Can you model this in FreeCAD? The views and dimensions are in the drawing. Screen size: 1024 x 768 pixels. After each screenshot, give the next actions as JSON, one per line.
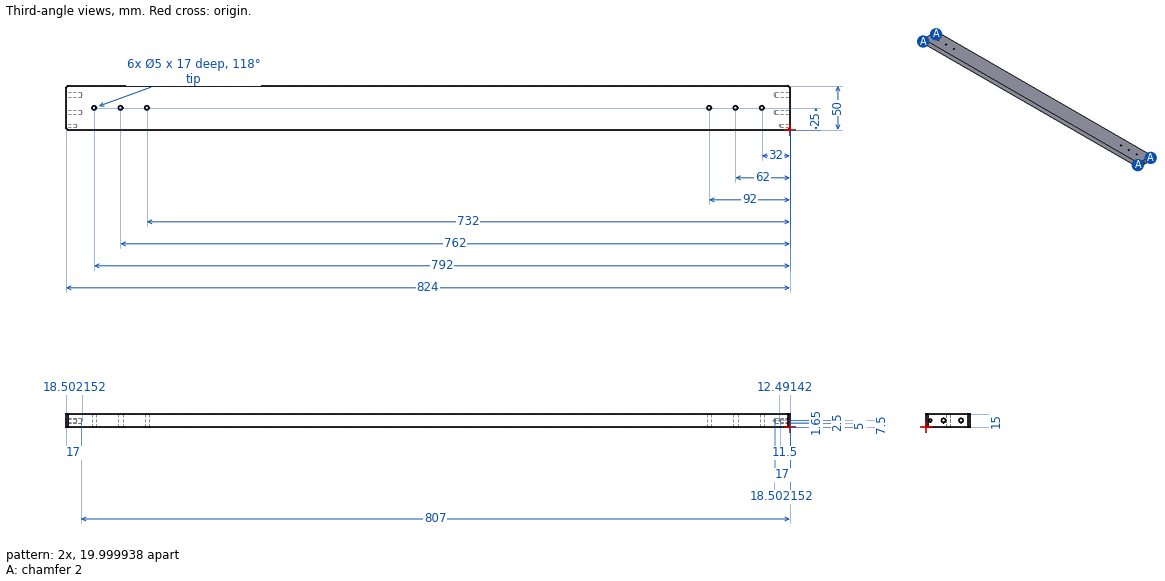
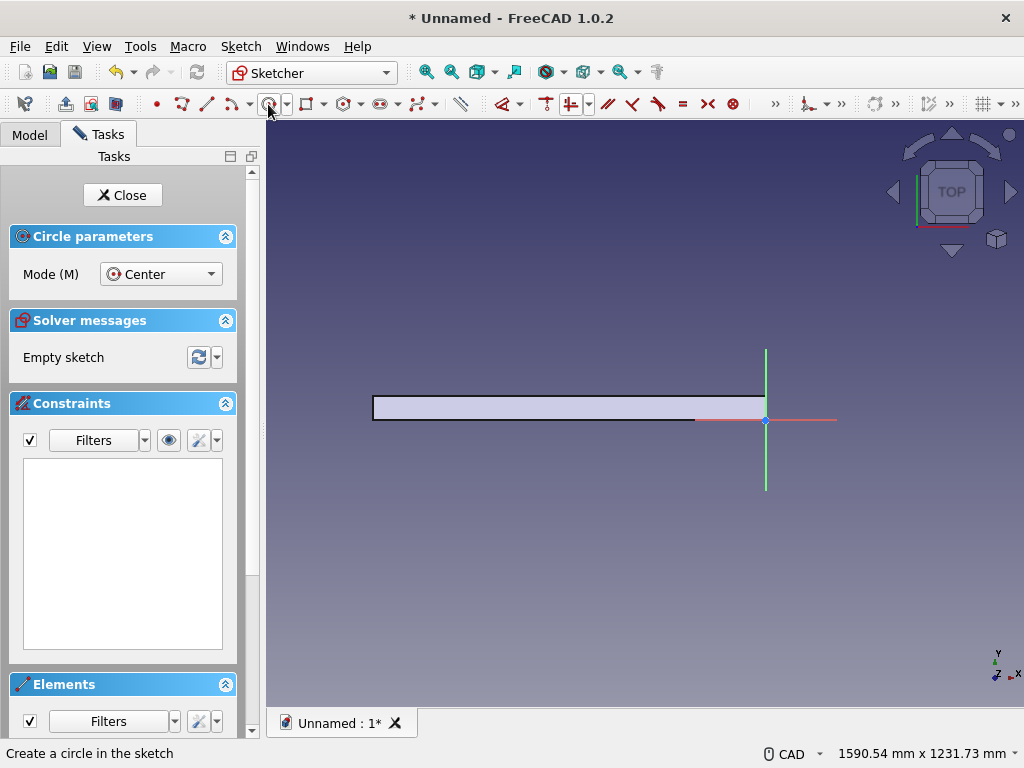
{"action": "scroll", "coordinate": [388, 408], "scroll_direction": "up", "scroll_amount": 15}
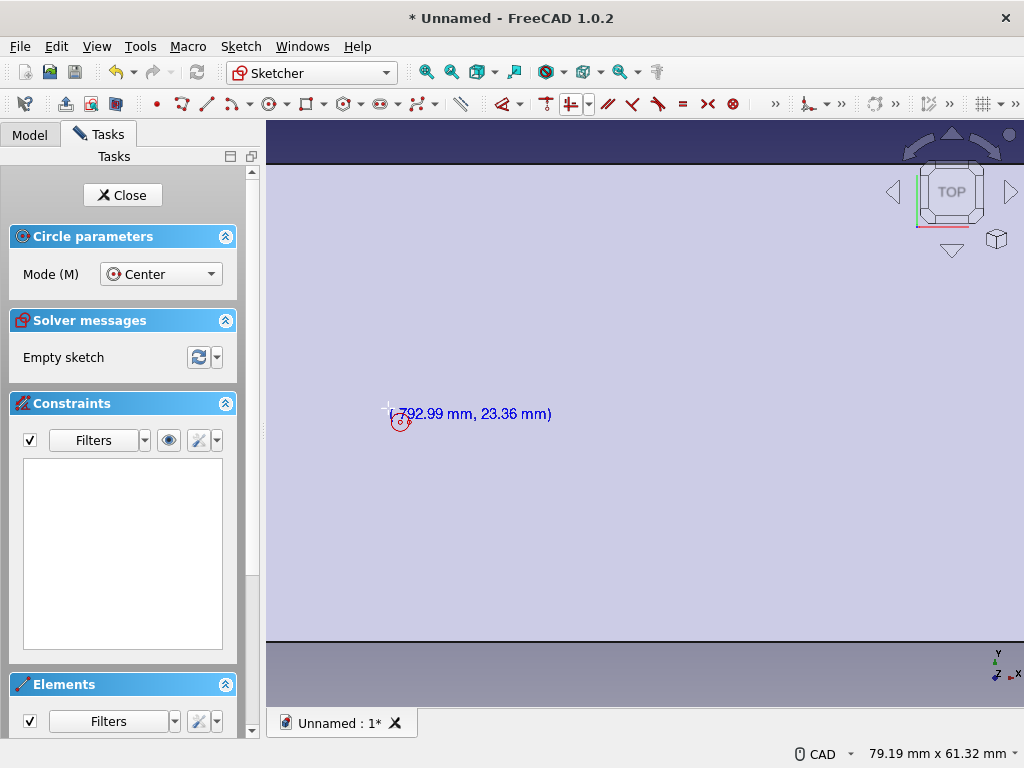
{"action": "scroll", "coordinate": [388, 408], "scroll_direction": "down", "scroll_amount": 15}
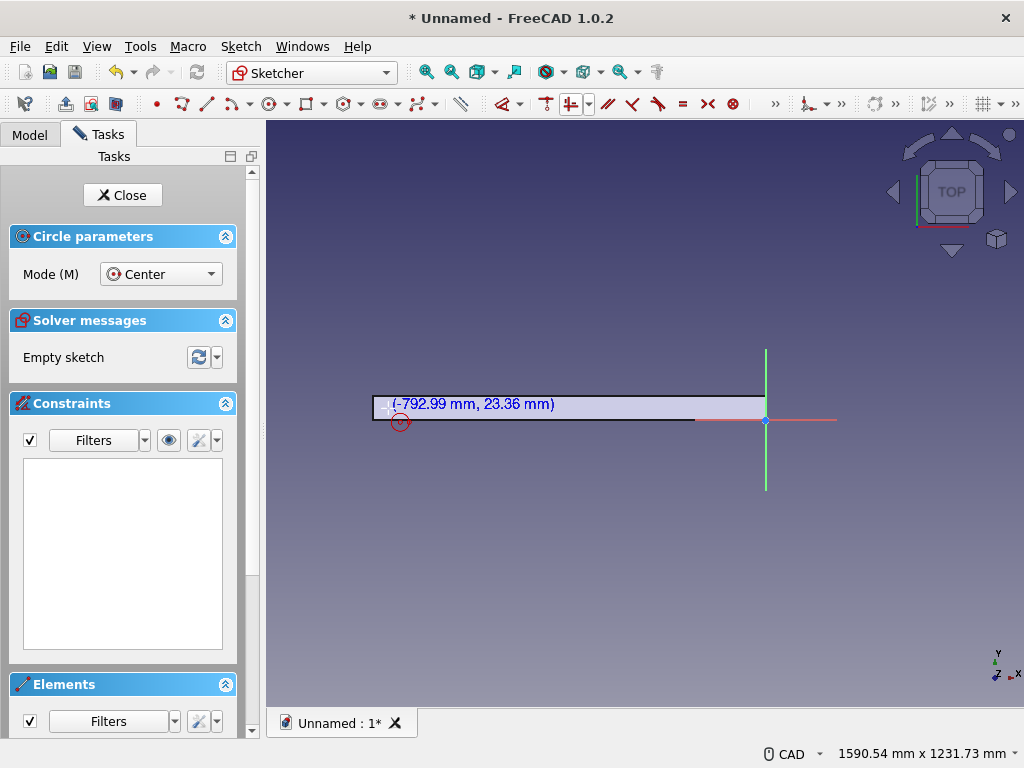
{"action": "scroll", "coordinate": [388, 408], "scroll_direction": "up", "scroll_amount": 2}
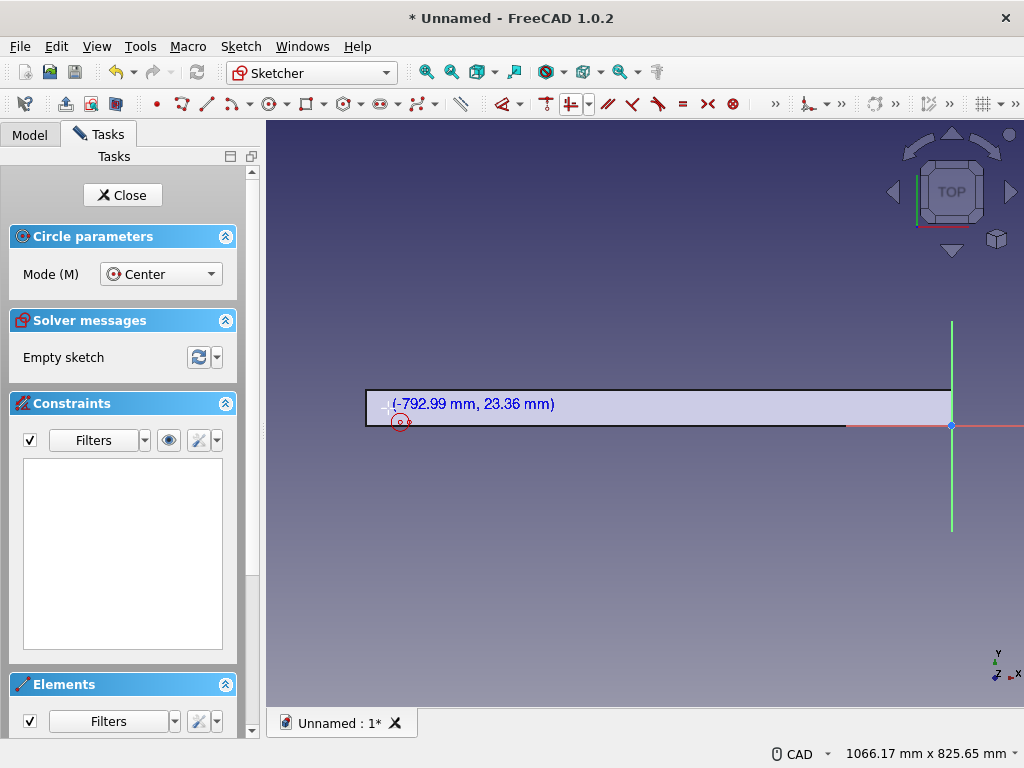
{"action": "left_click", "coordinate": [389, 408]}
{"action": "mouse_move", "coordinate": [390, 407]}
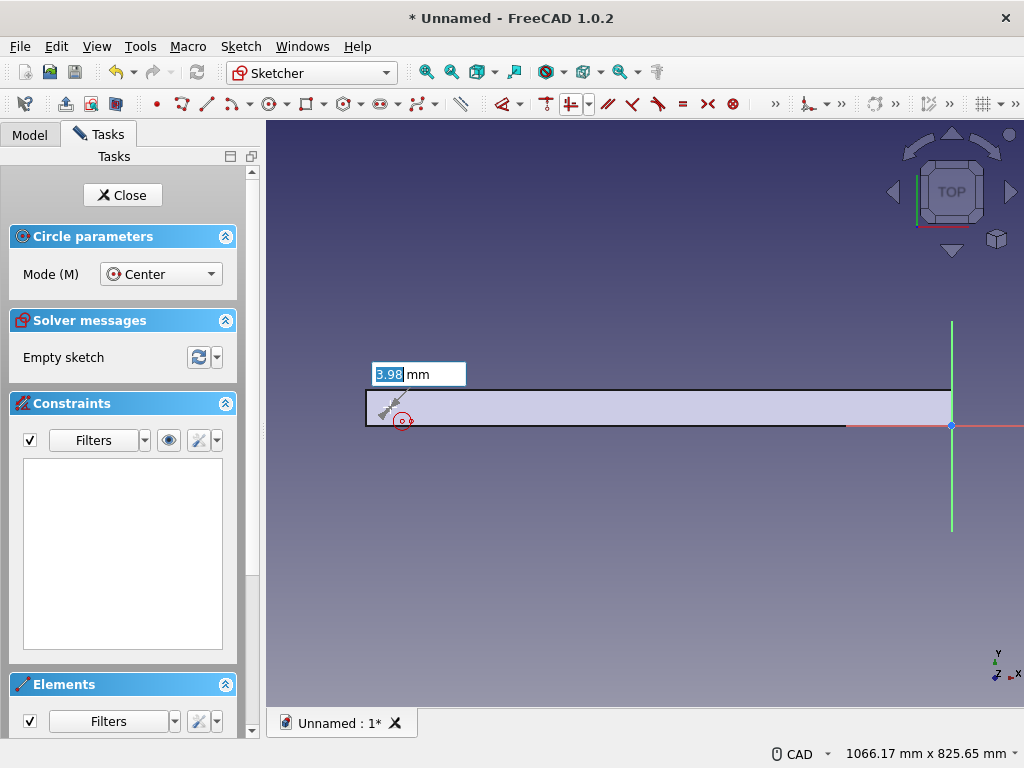
{"action": "type", "text": "5"}
{"action": "key", "text": "Return"}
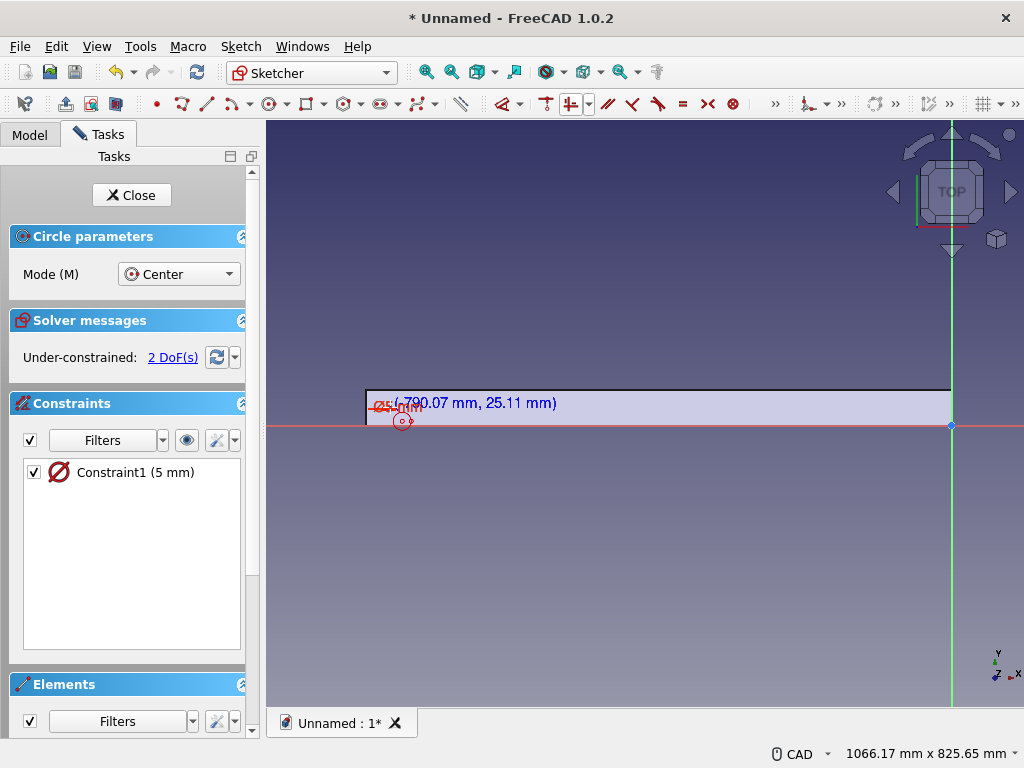
{"action": "scroll", "coordinate": [388, 408], "scroll_direction": "down", "scroll_amount": 2}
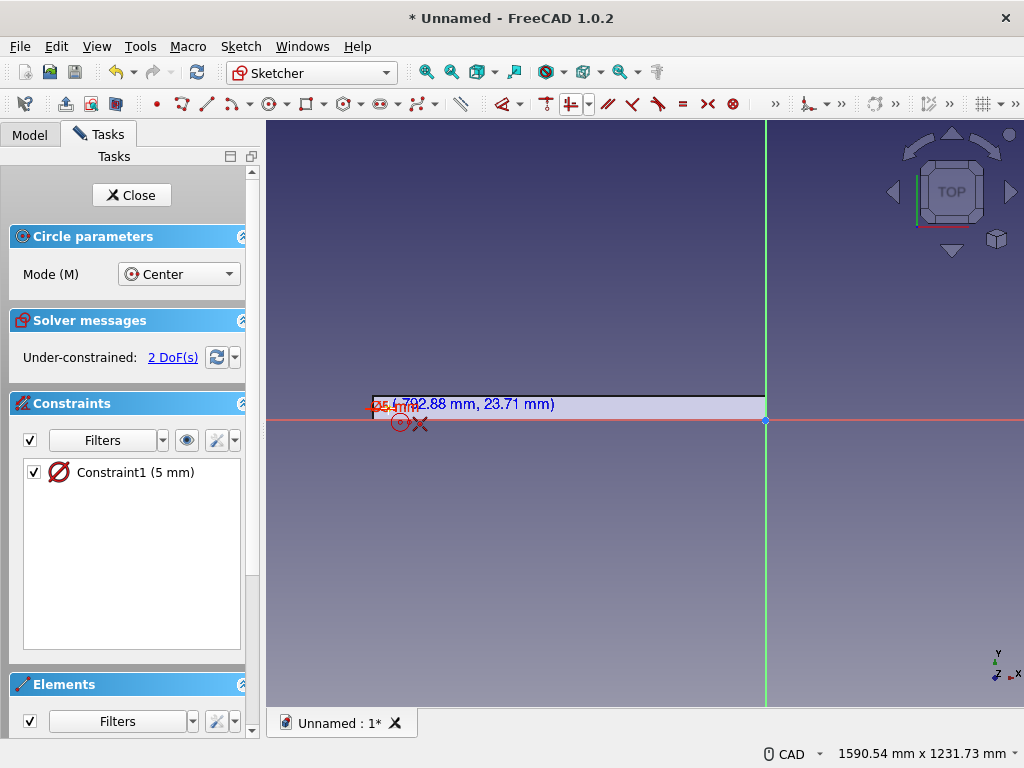
{"action": "scroll", "coordinate": [751, 408], "scroll_direction": "up", "scroll_amount": 15}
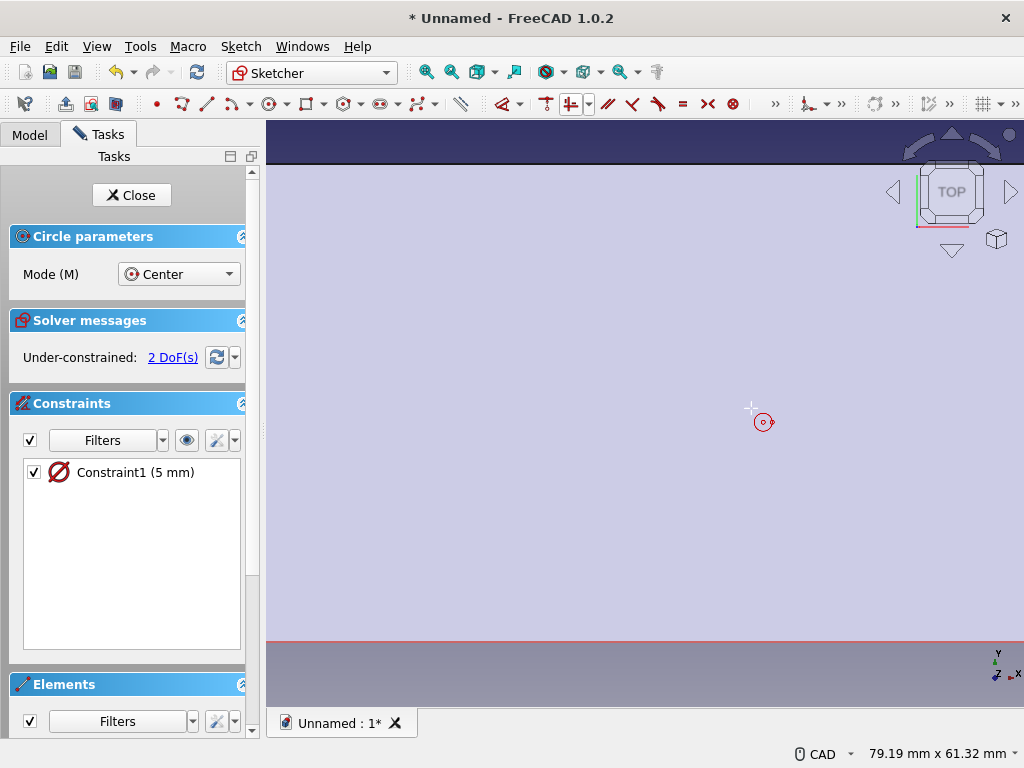
{"action": "scroll", "coordinate": [752, 408], "scroll_direction": "down", "scroll_amount": 15}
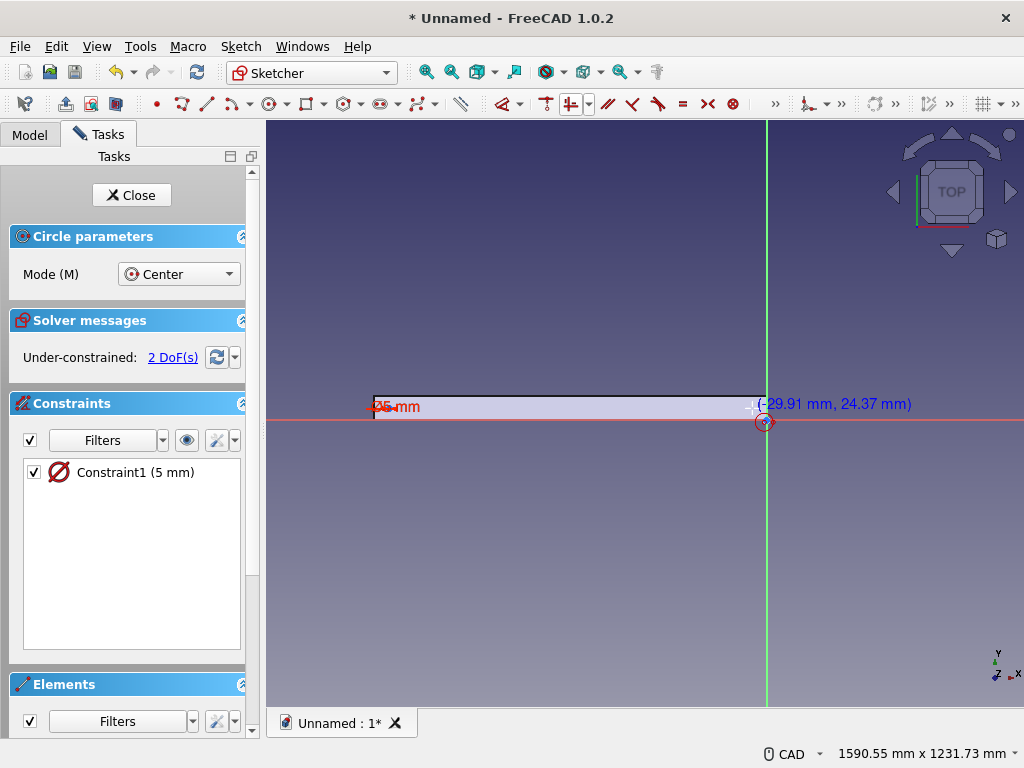
{"action": "scroll", "coordinate": [752, 408], "scroll_direction": "up", "scroll_amount": 2}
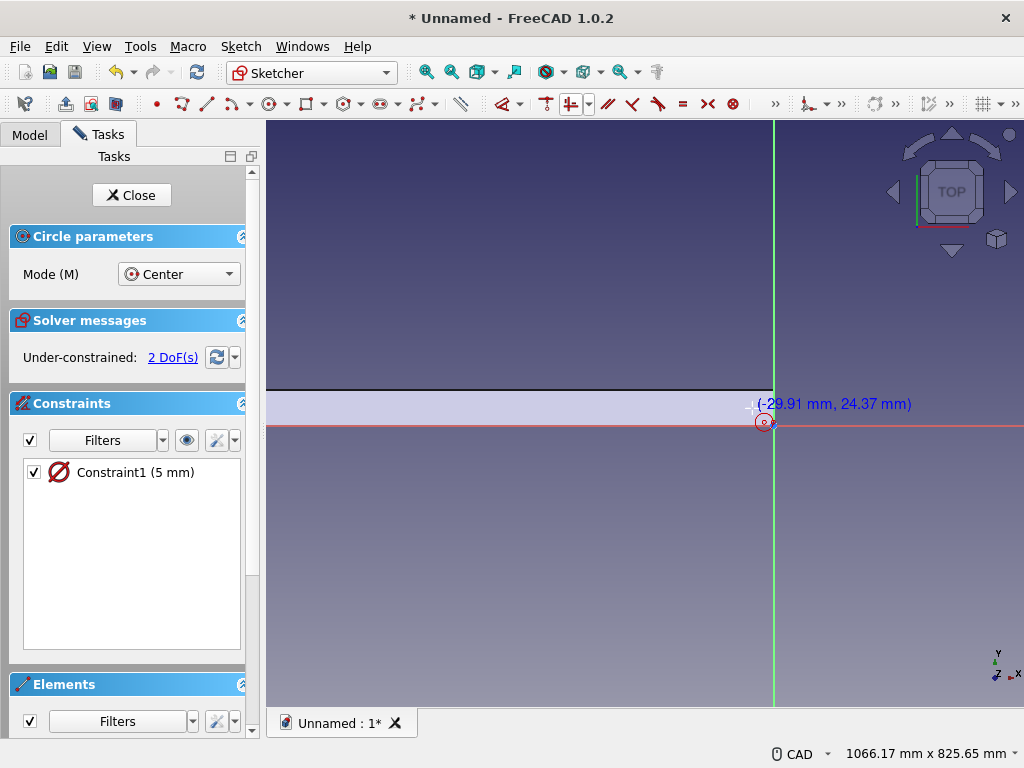
{"action": "left_click", "coordinate": [751, 408]}
{"action": "mouse_move", "coordinate": [752, 407]}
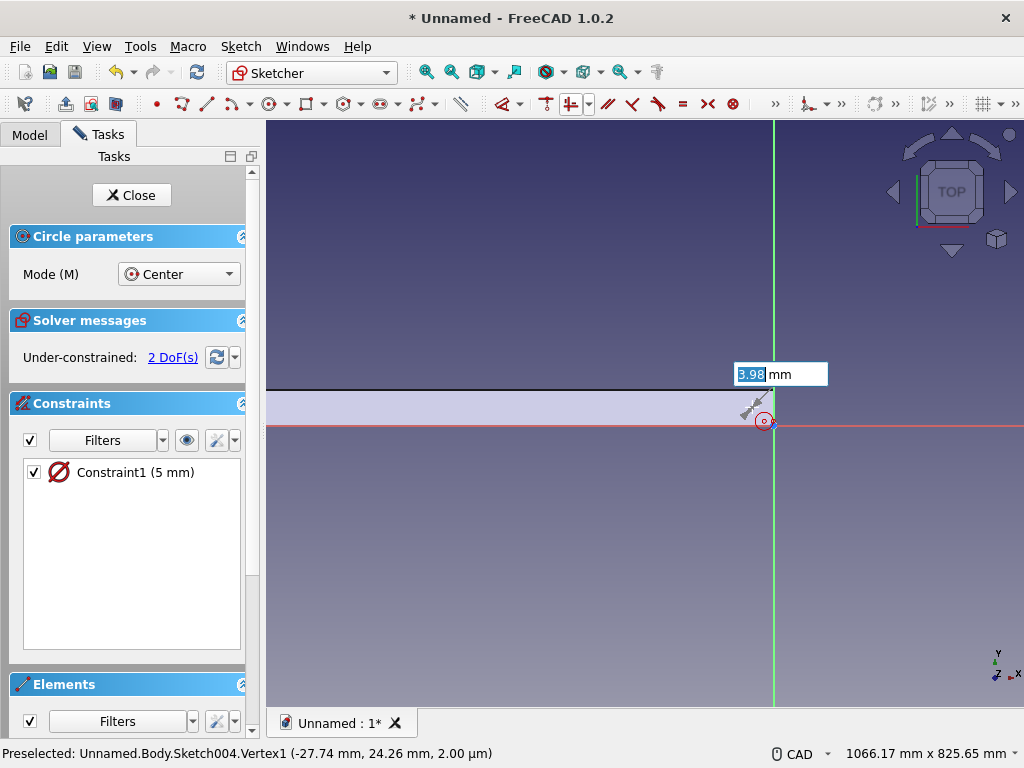
{"action": "type", "text": "5"}
{"action": "key", "text": "Return"}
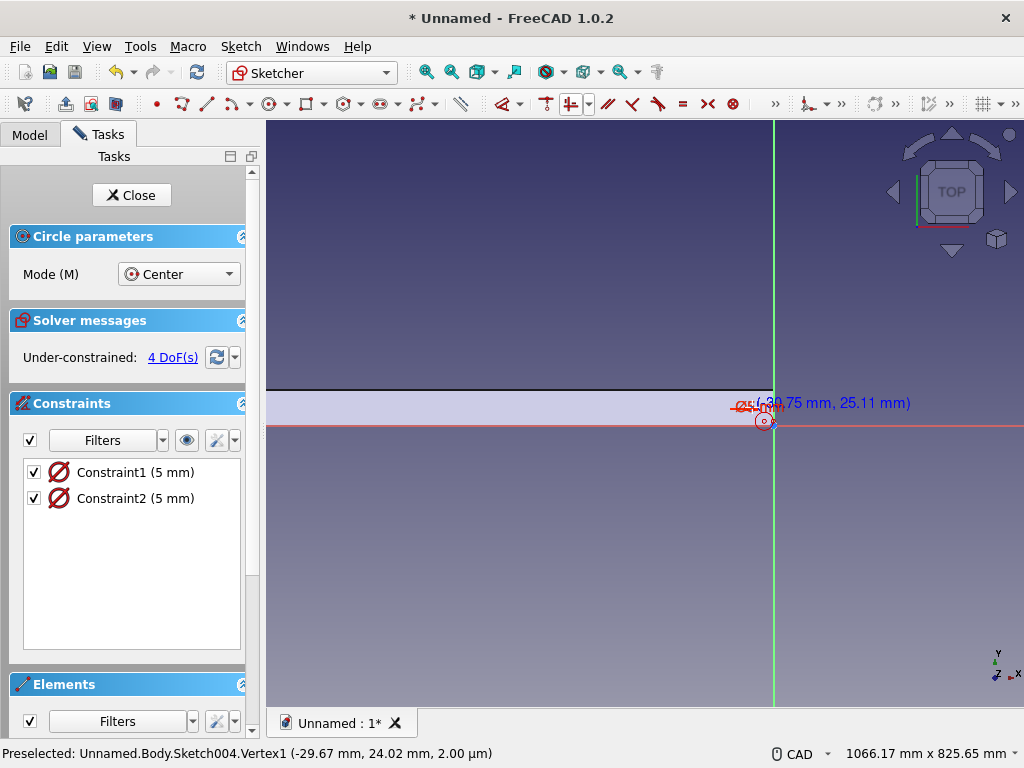
{"action": "scroll", "coordinate": [730, 408], "scroll_direction": "up", "scroll_amount": 13}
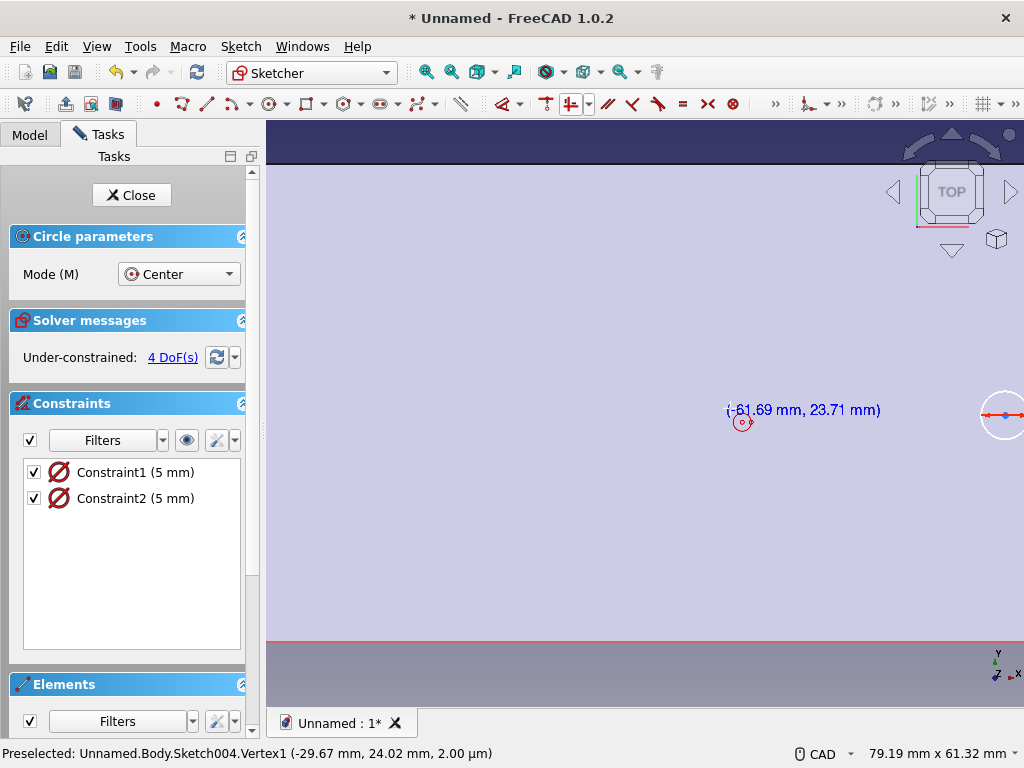
{"action": "scroll", "coordinate": [737, 408], "scroll_direction": "down", "scroll_amount": 15}